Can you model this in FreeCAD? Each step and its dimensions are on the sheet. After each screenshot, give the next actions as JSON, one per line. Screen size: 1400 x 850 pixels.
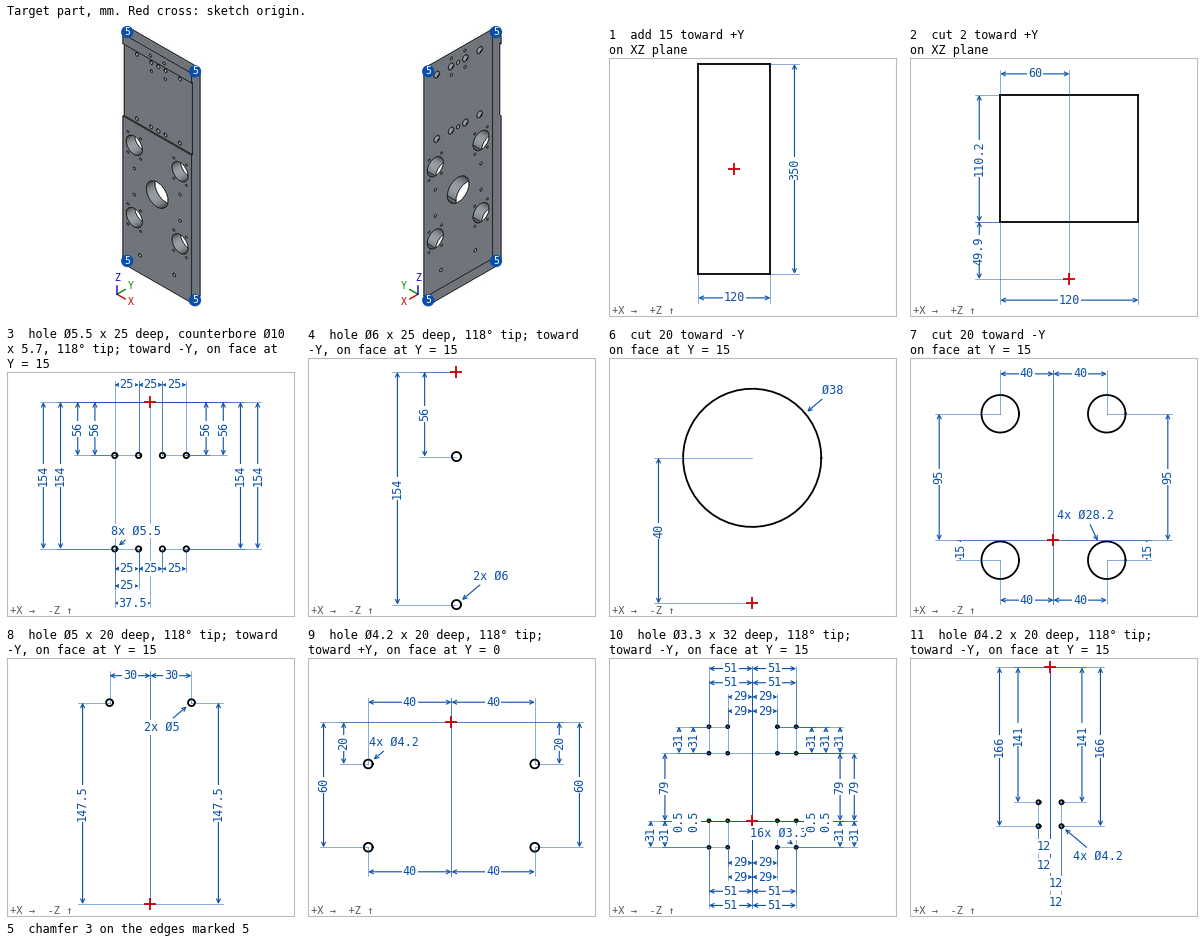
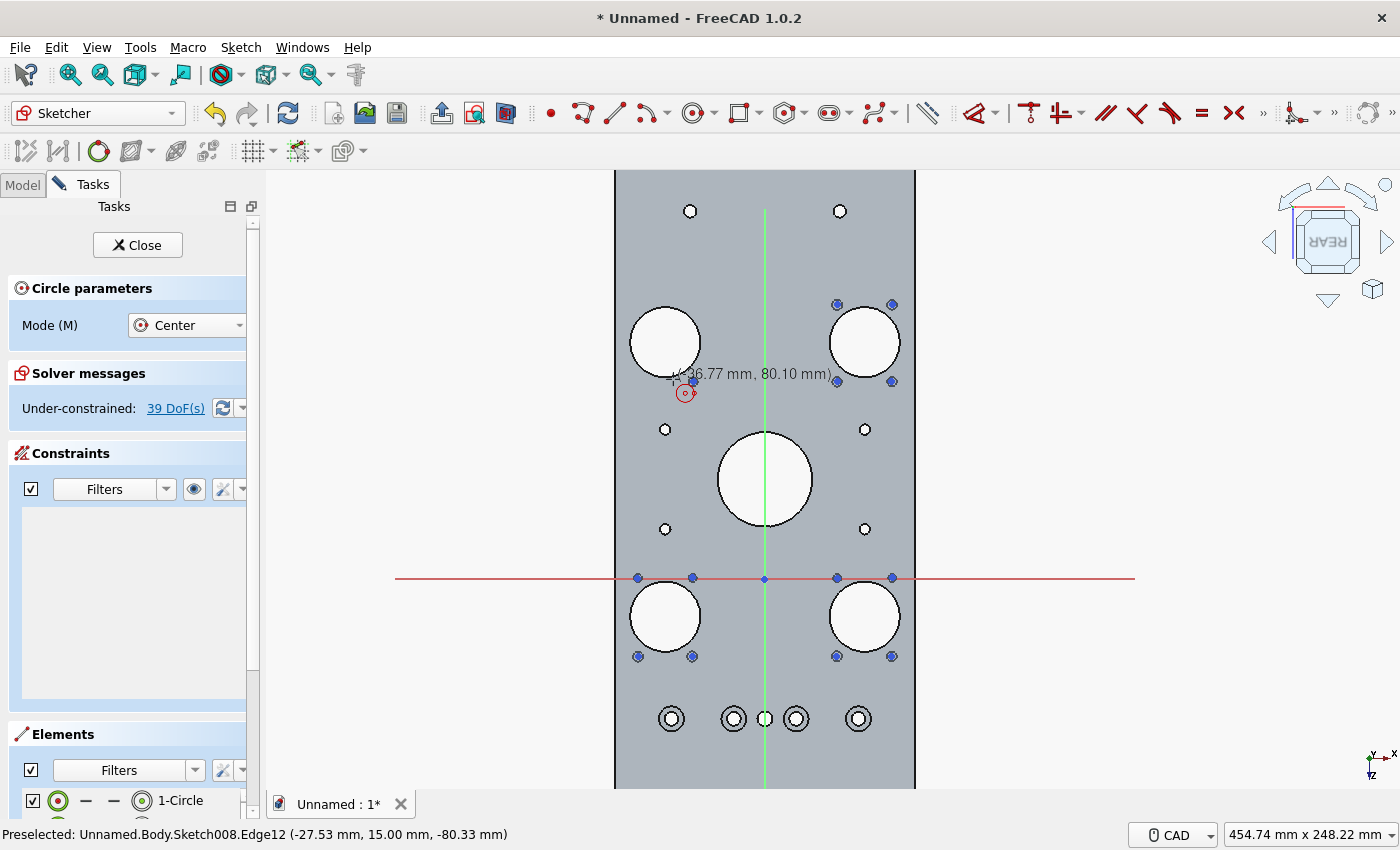
{"action": "left_click", "coordinate": [638, 381]}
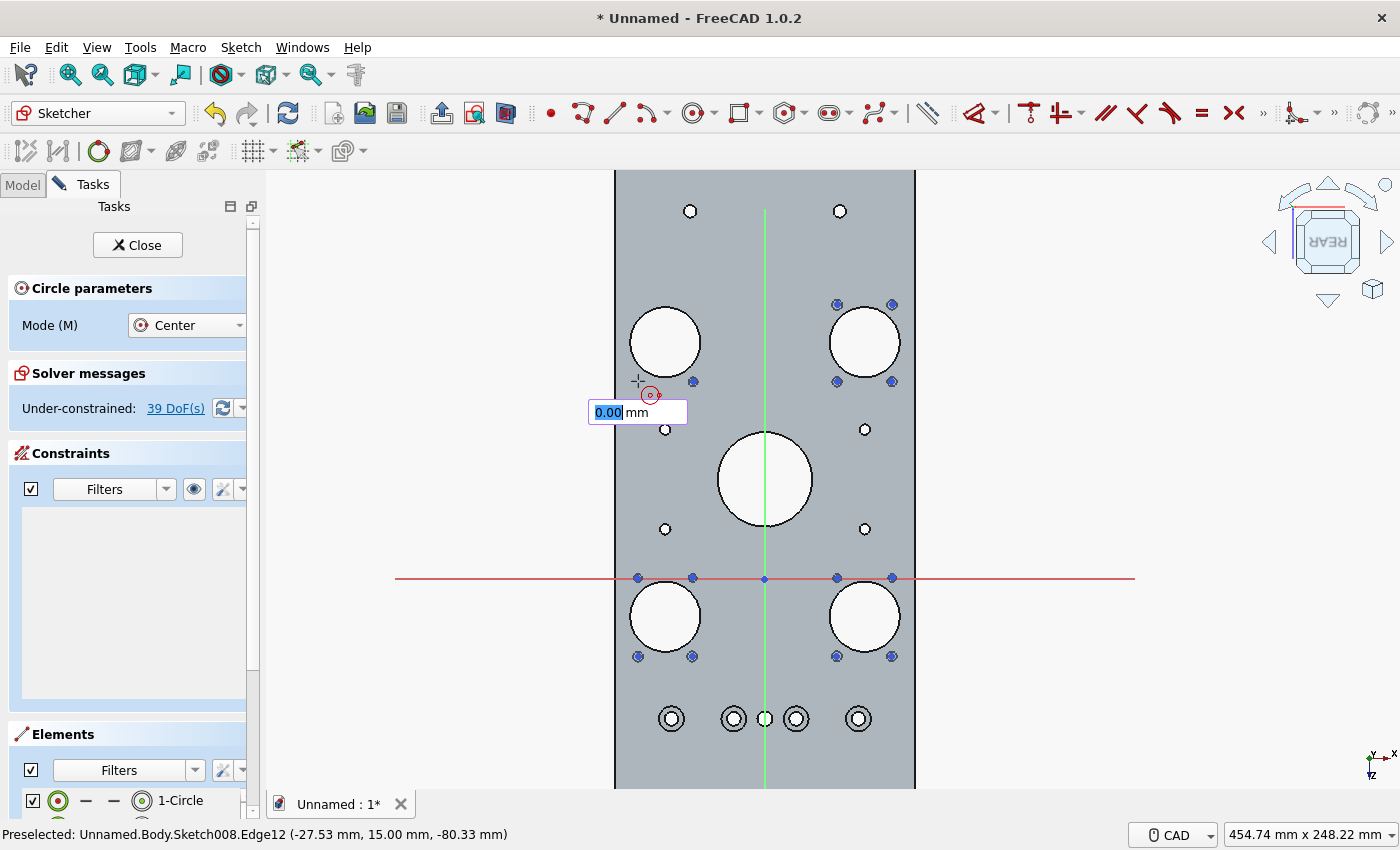
{"action": "scroll", "coordinate": [641, 378], "scroll_direction": "up", "scroll_amount": 7}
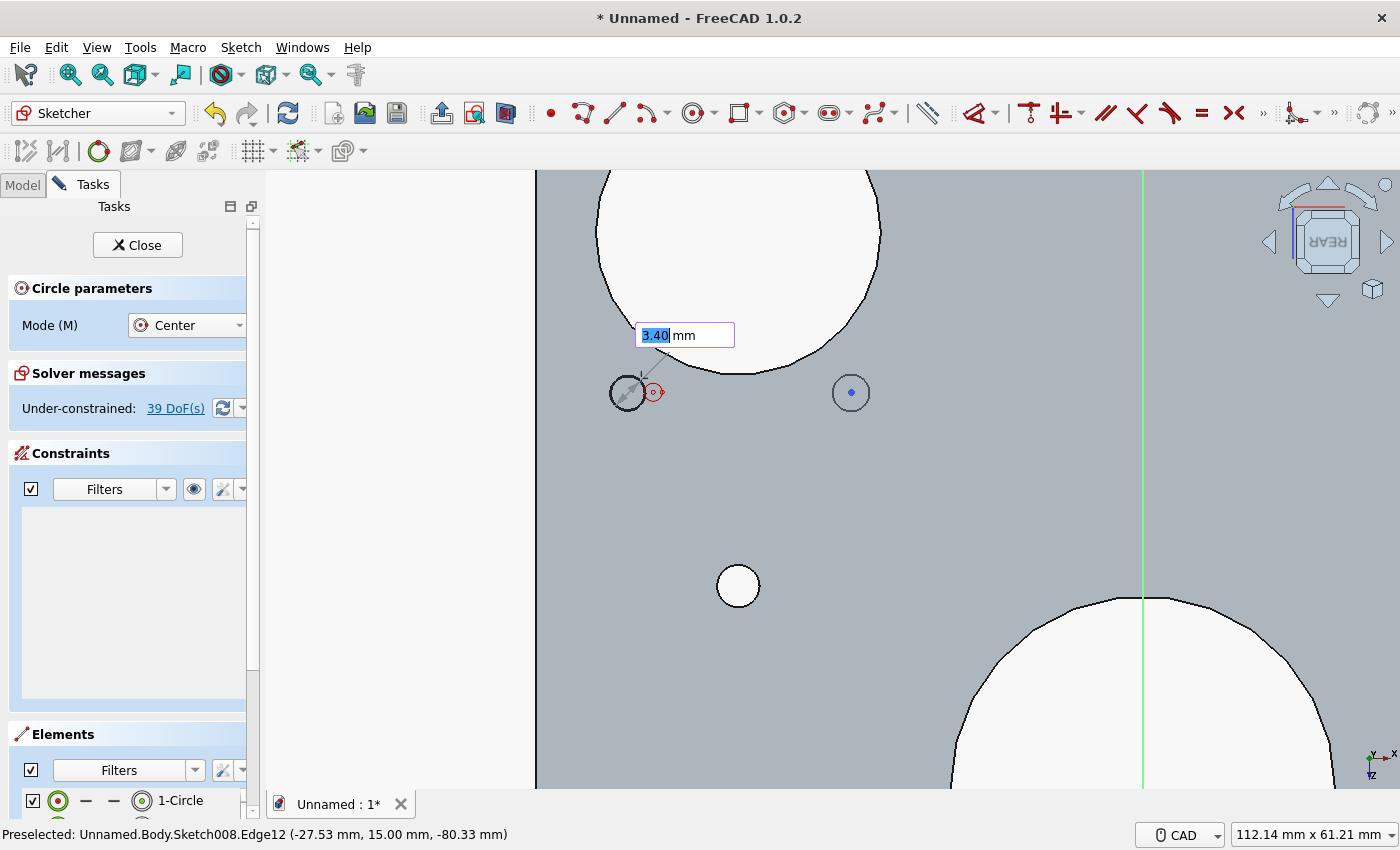
{"action": "left_click", "coordinate": [639, 377]}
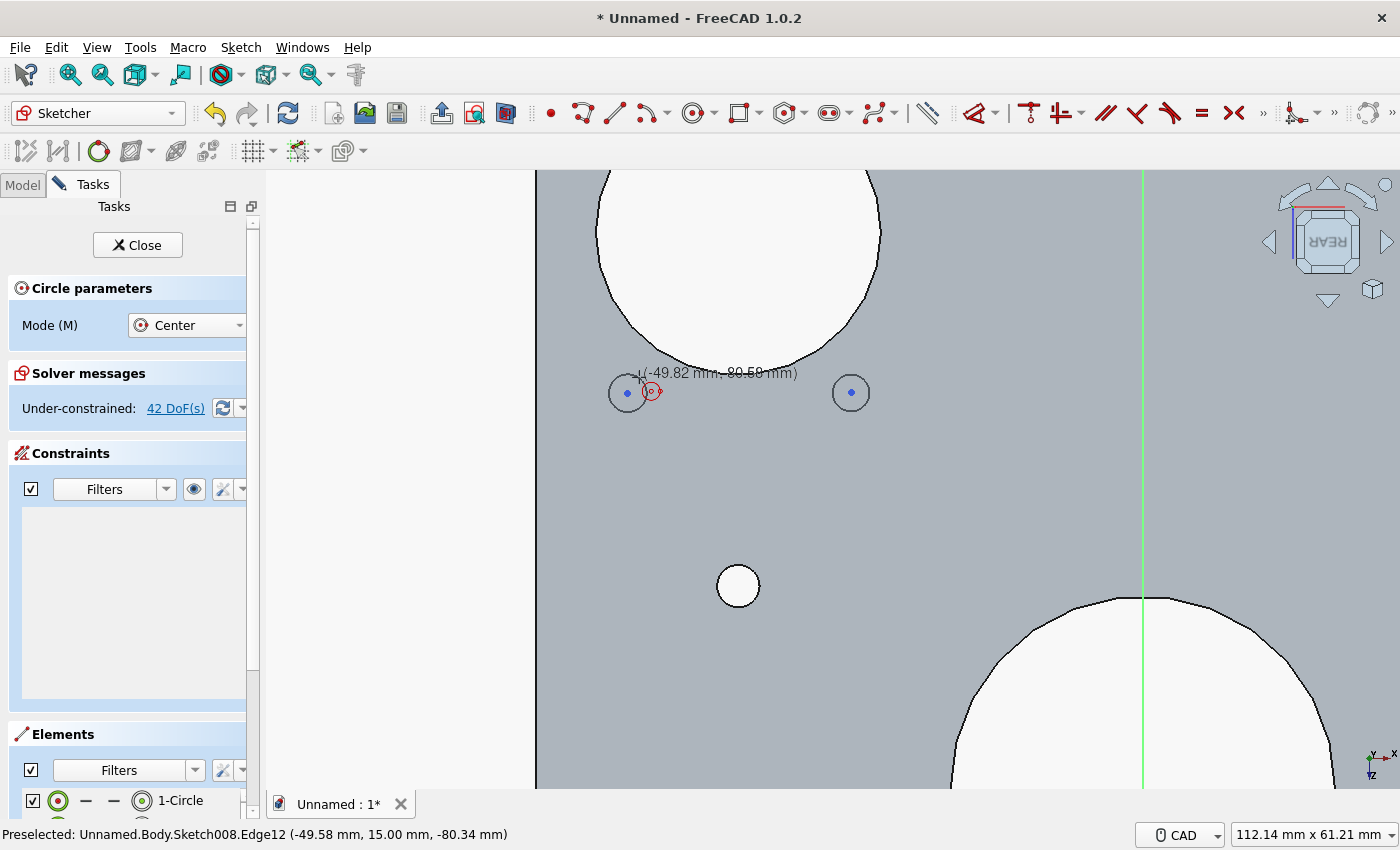
{"action": "scroll", "coordinate": [641, 378], "scroll_direction": "down", "scroll_amount": 7}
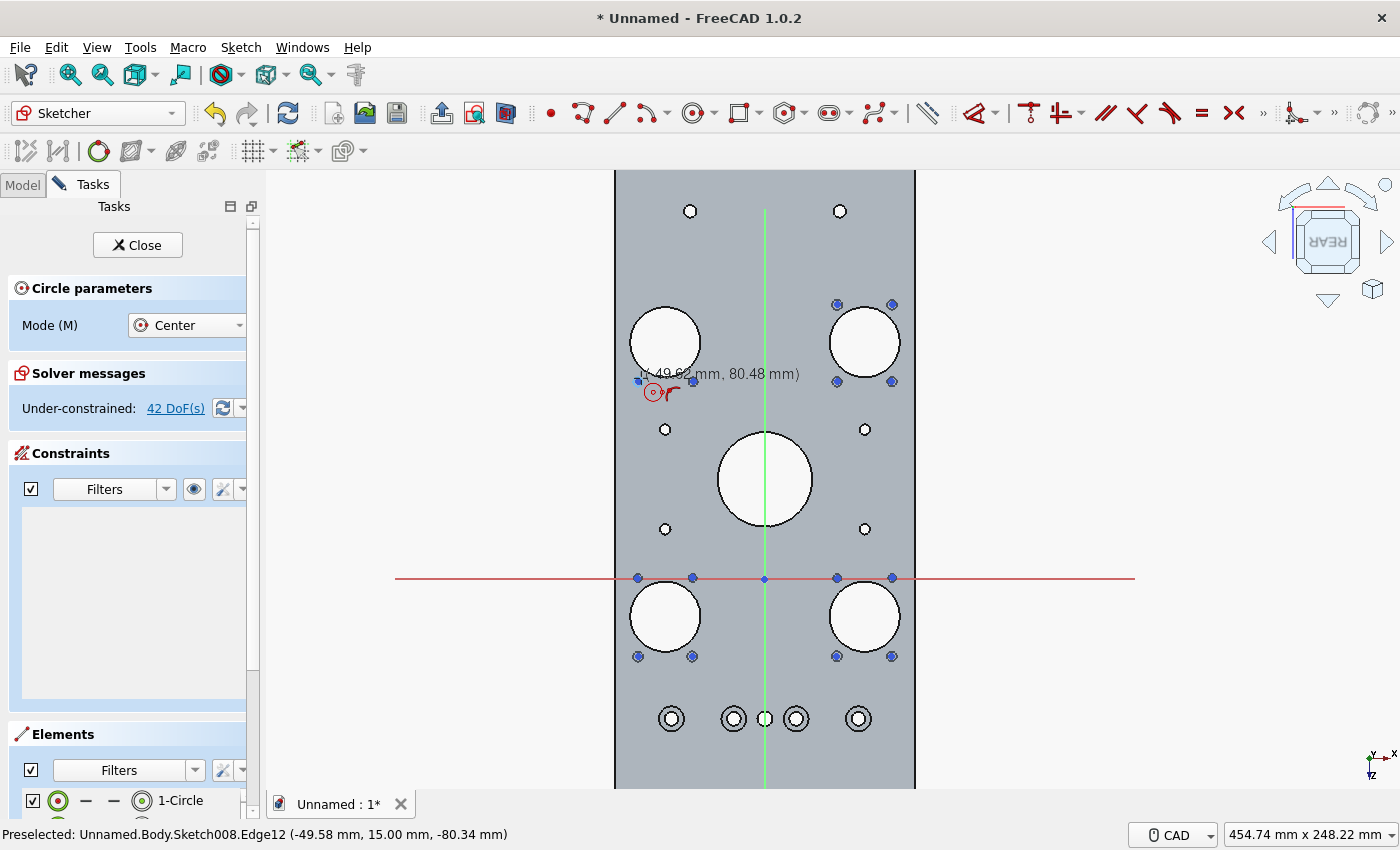
{"action": "scroll", "coordinate": [693, 304], "scroll_direction": "up", "scroll_amount": 9}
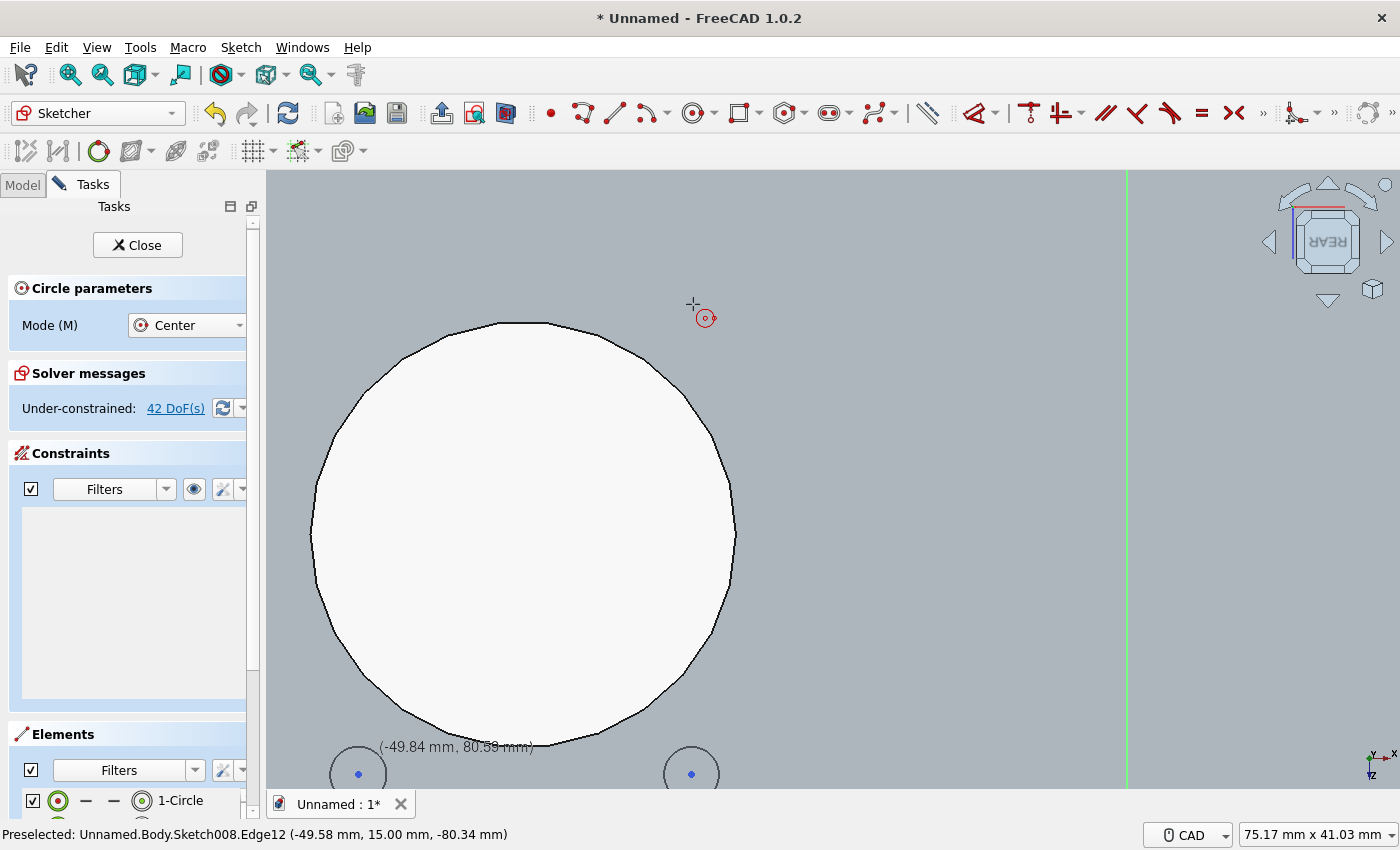
{"action": "scroll", "coordinate": [693, 304], "scroll_direction": "down", "scroll_amount": 9}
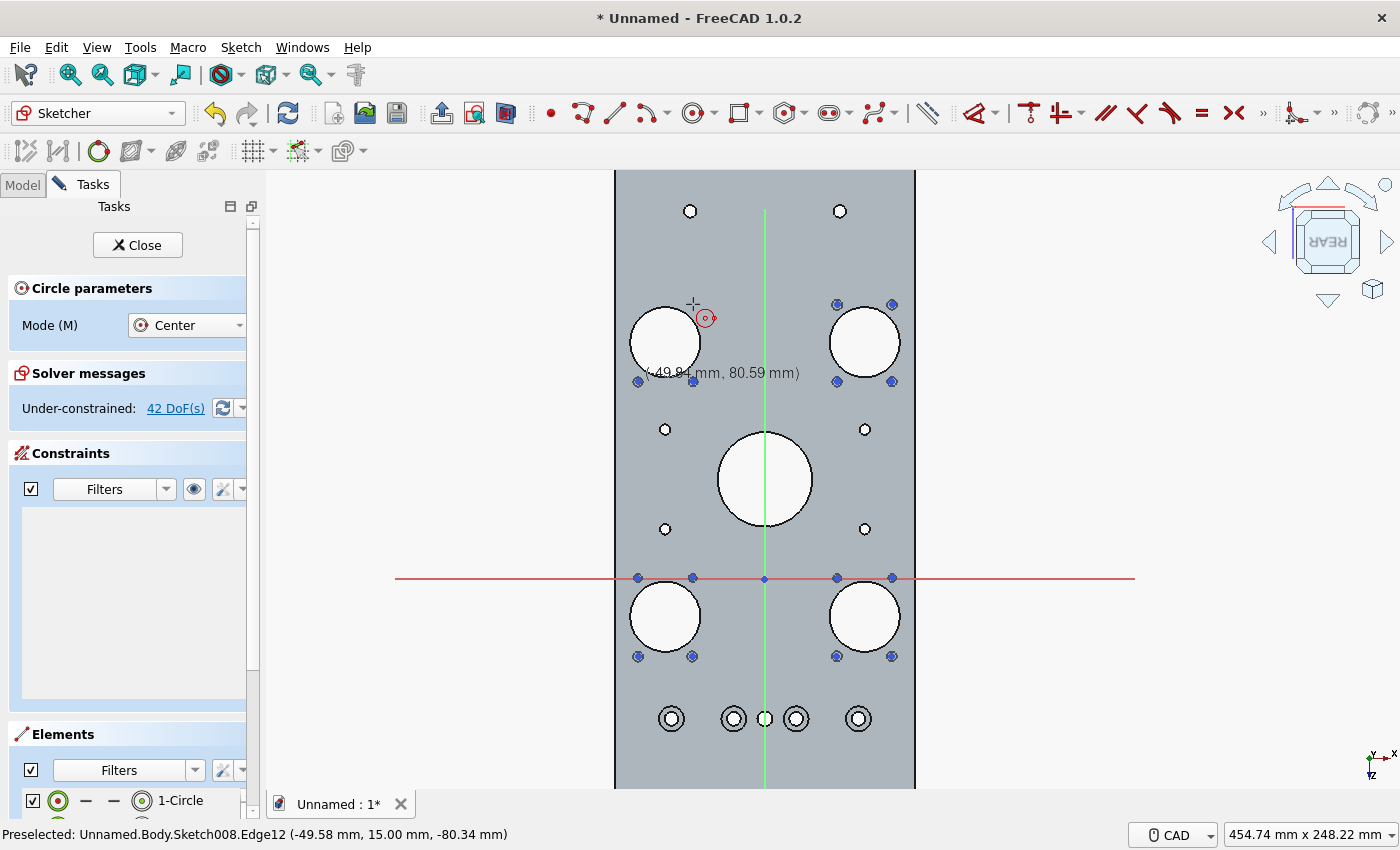
{"action": "left_click", "coordinate": [693, 304]}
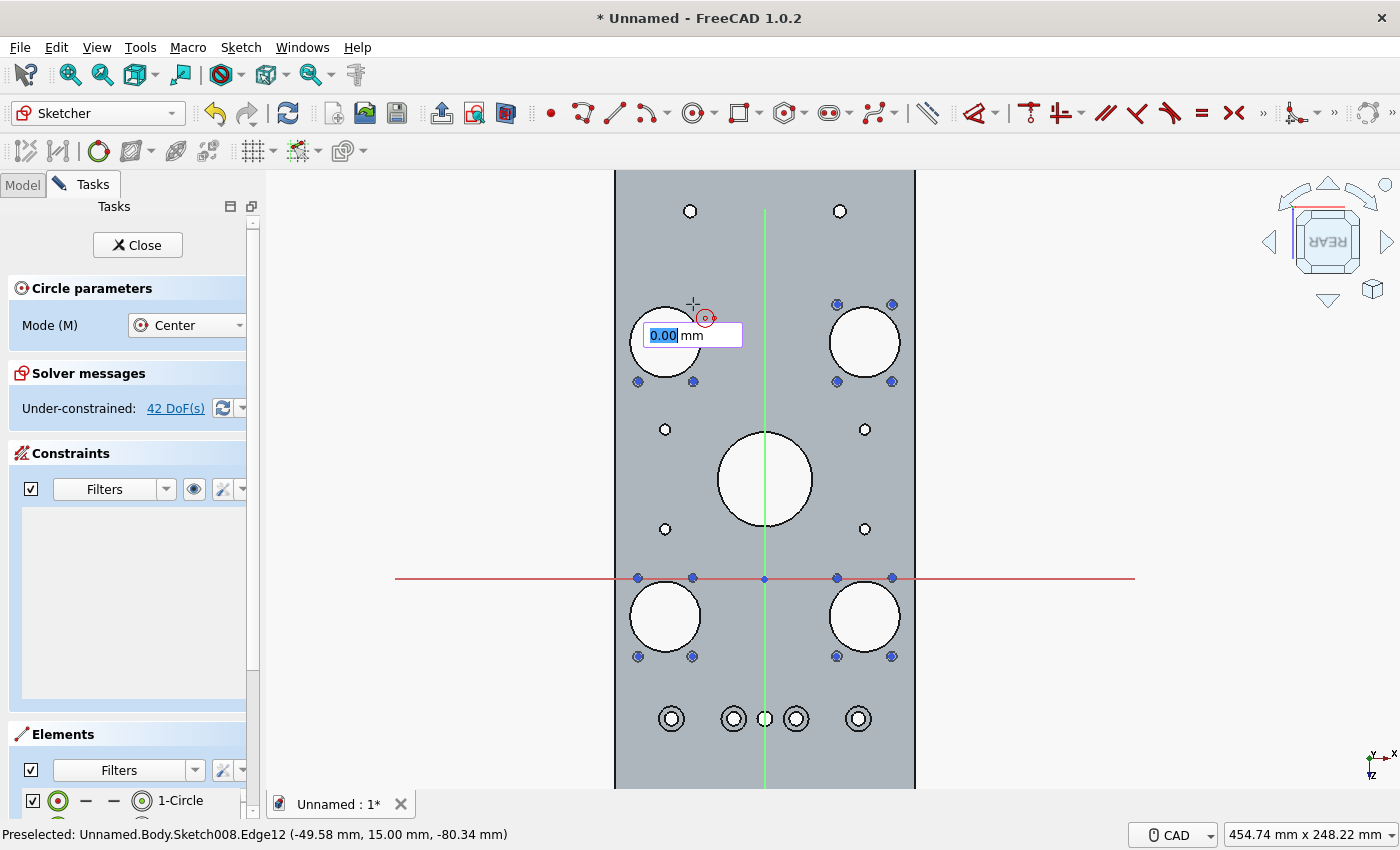
{"action": "scroll", "coordinate": [696, 301], "scroll_direction": "up", "scroll_amount": 7}